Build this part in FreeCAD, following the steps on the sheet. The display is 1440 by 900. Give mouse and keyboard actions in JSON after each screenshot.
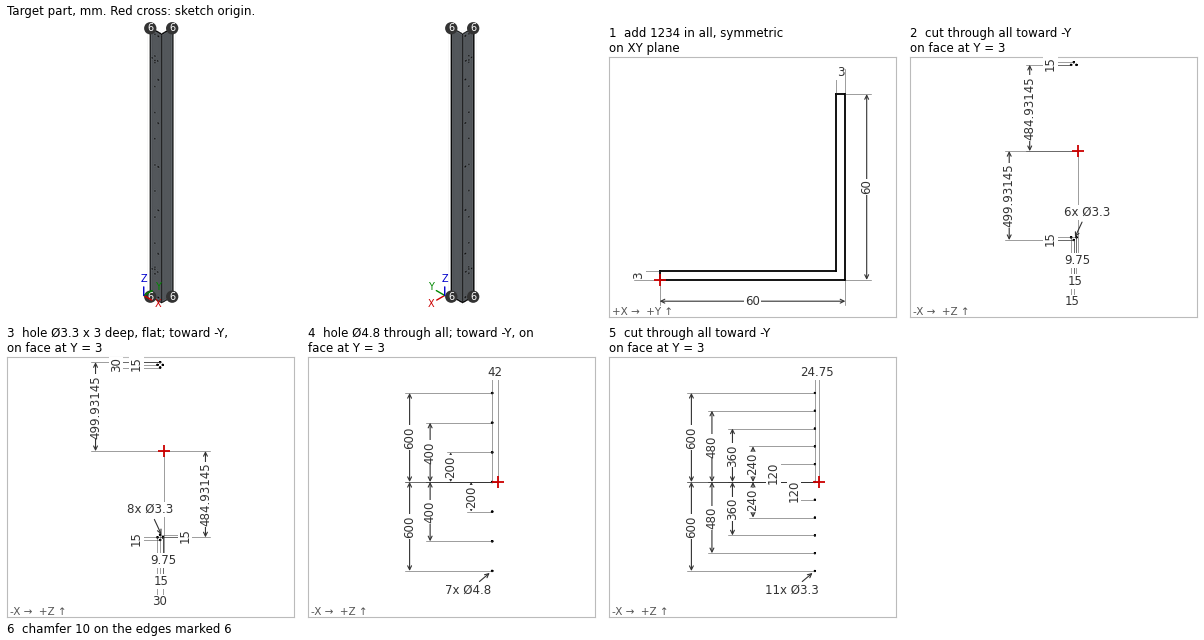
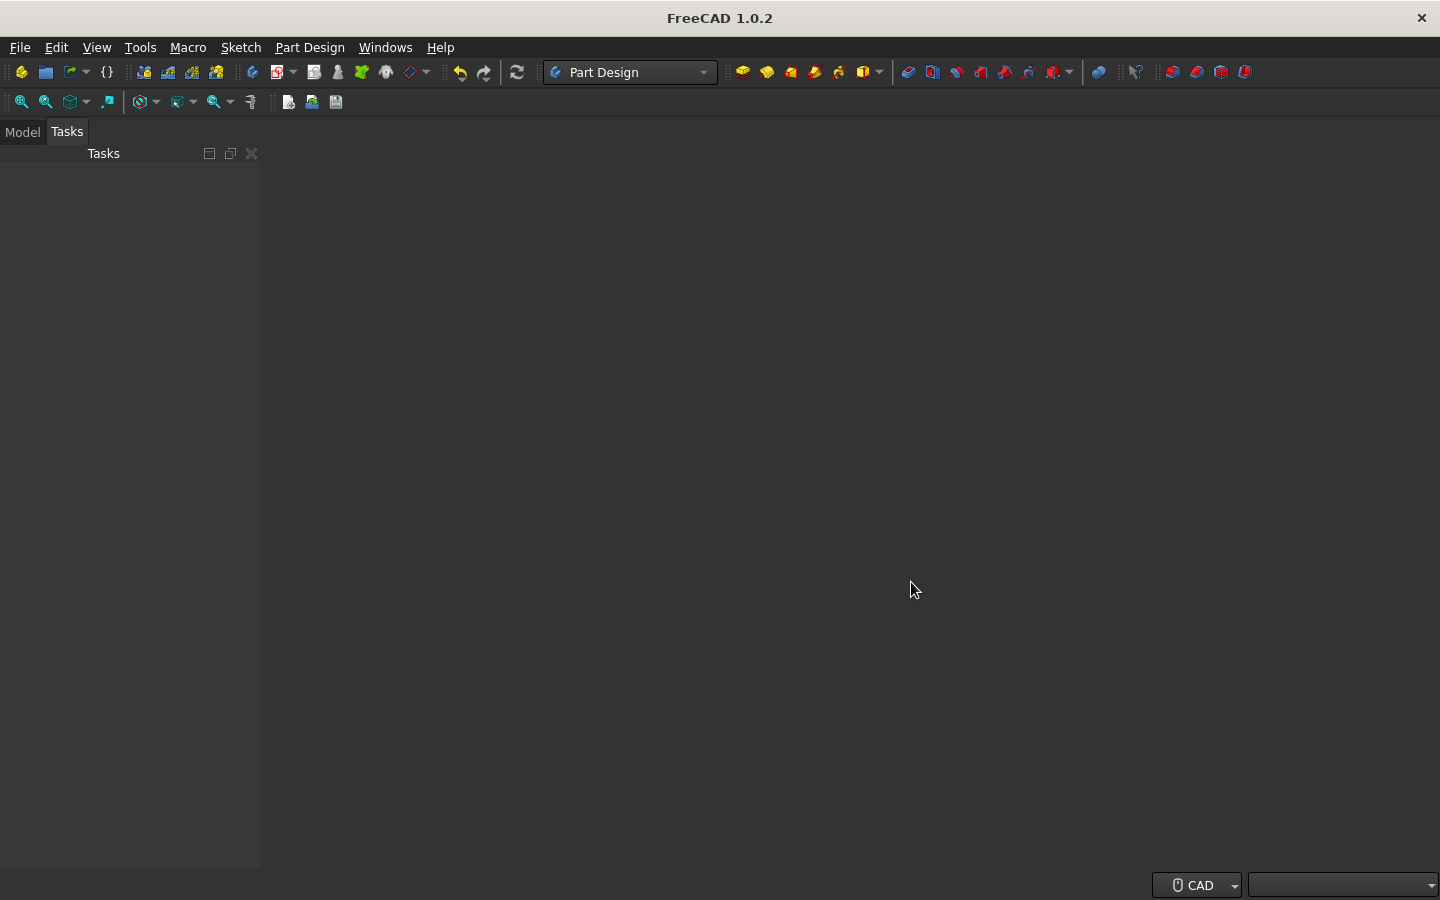
{"action": "left_click", "coordinate": [288, 102]}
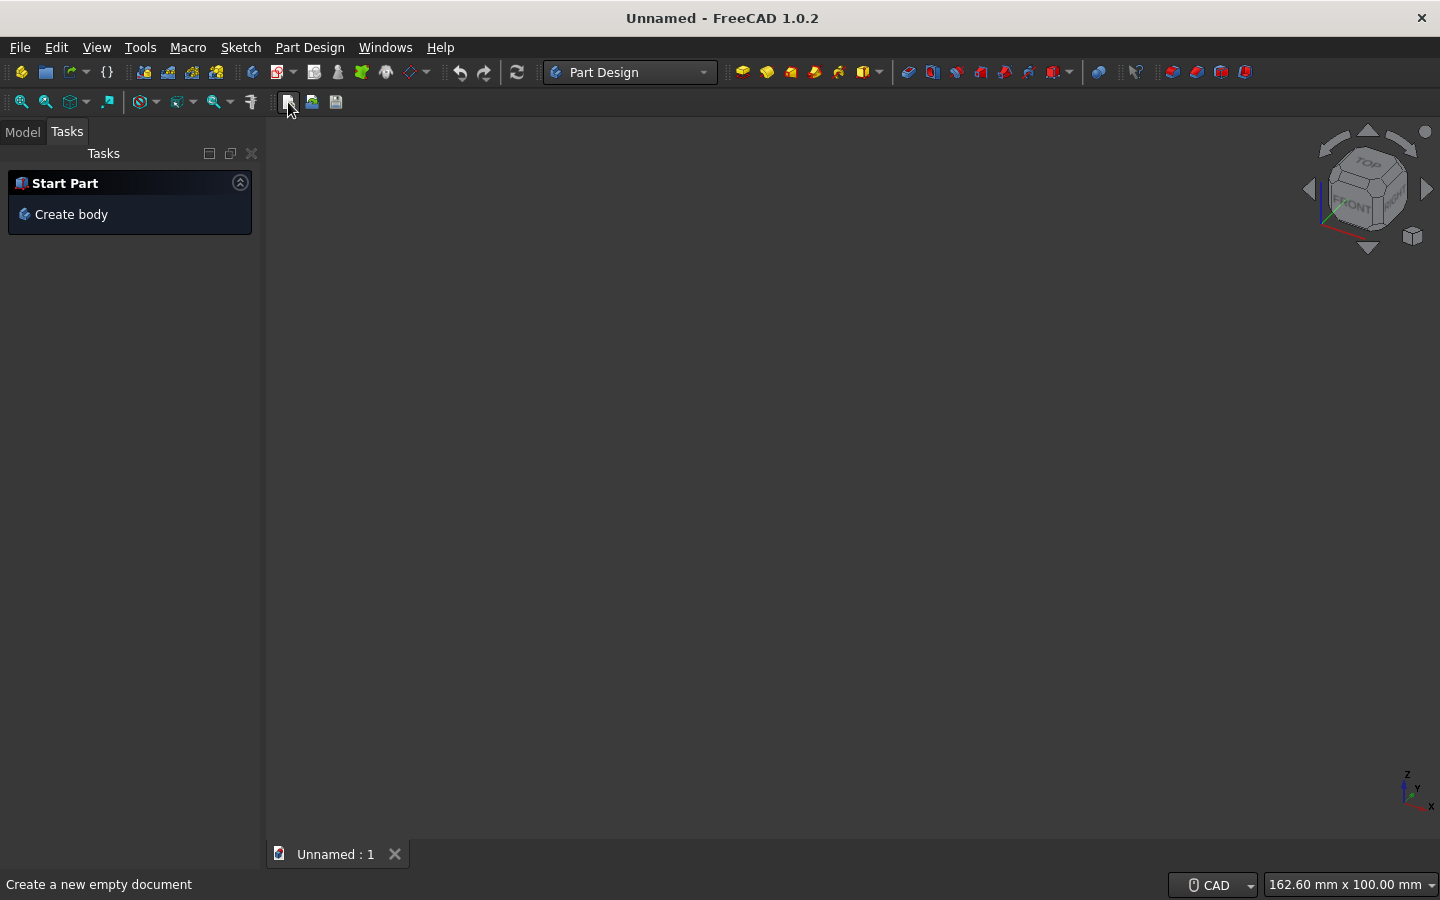
{"action": "left_click", "coordinate": [278, 72]}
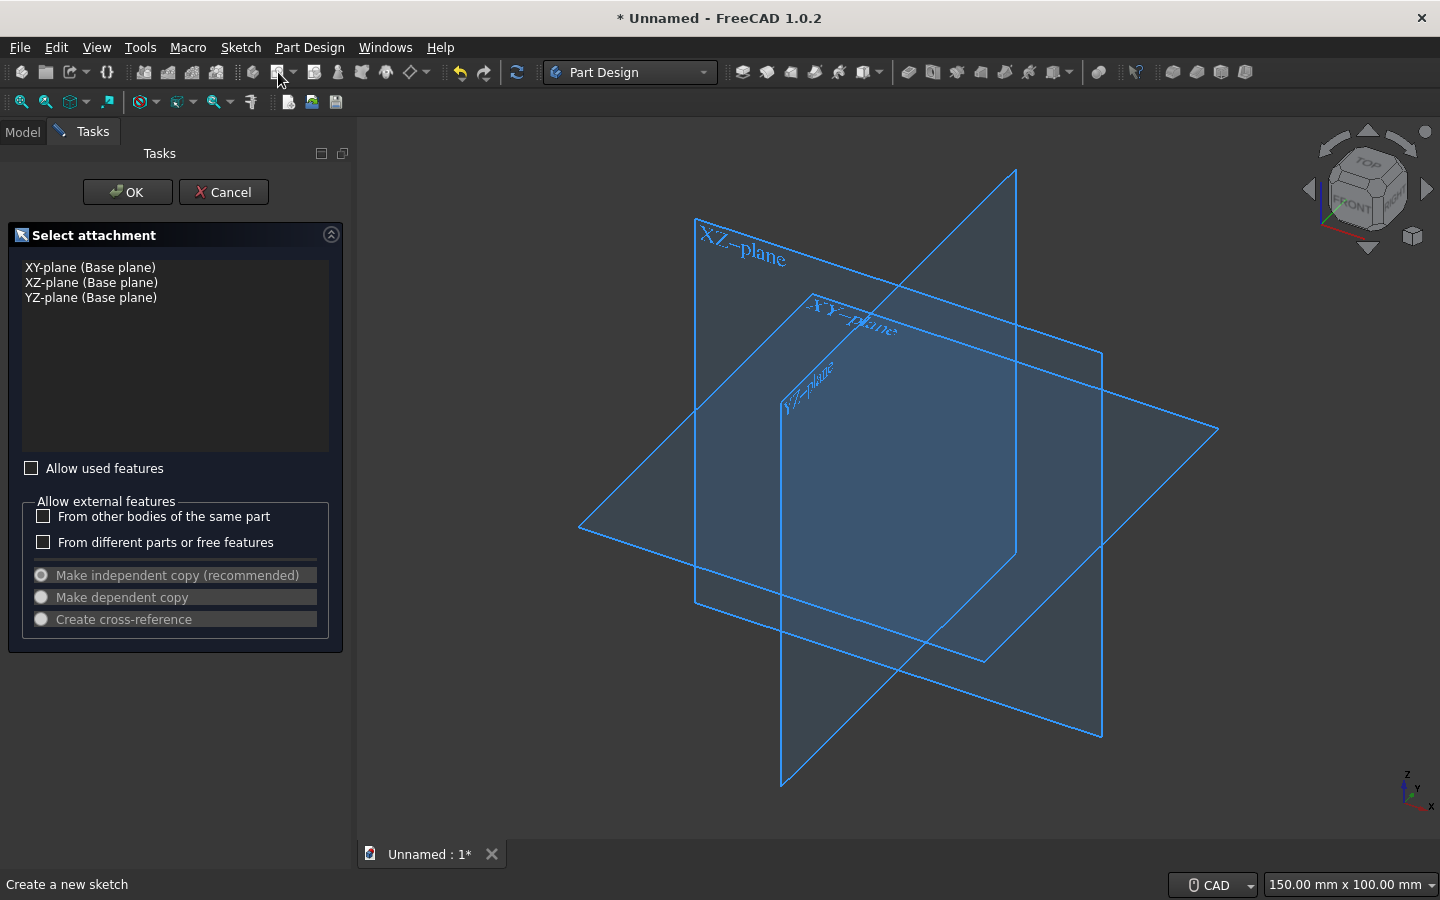
{"action": "left_click", "coordinate": [82, 268]}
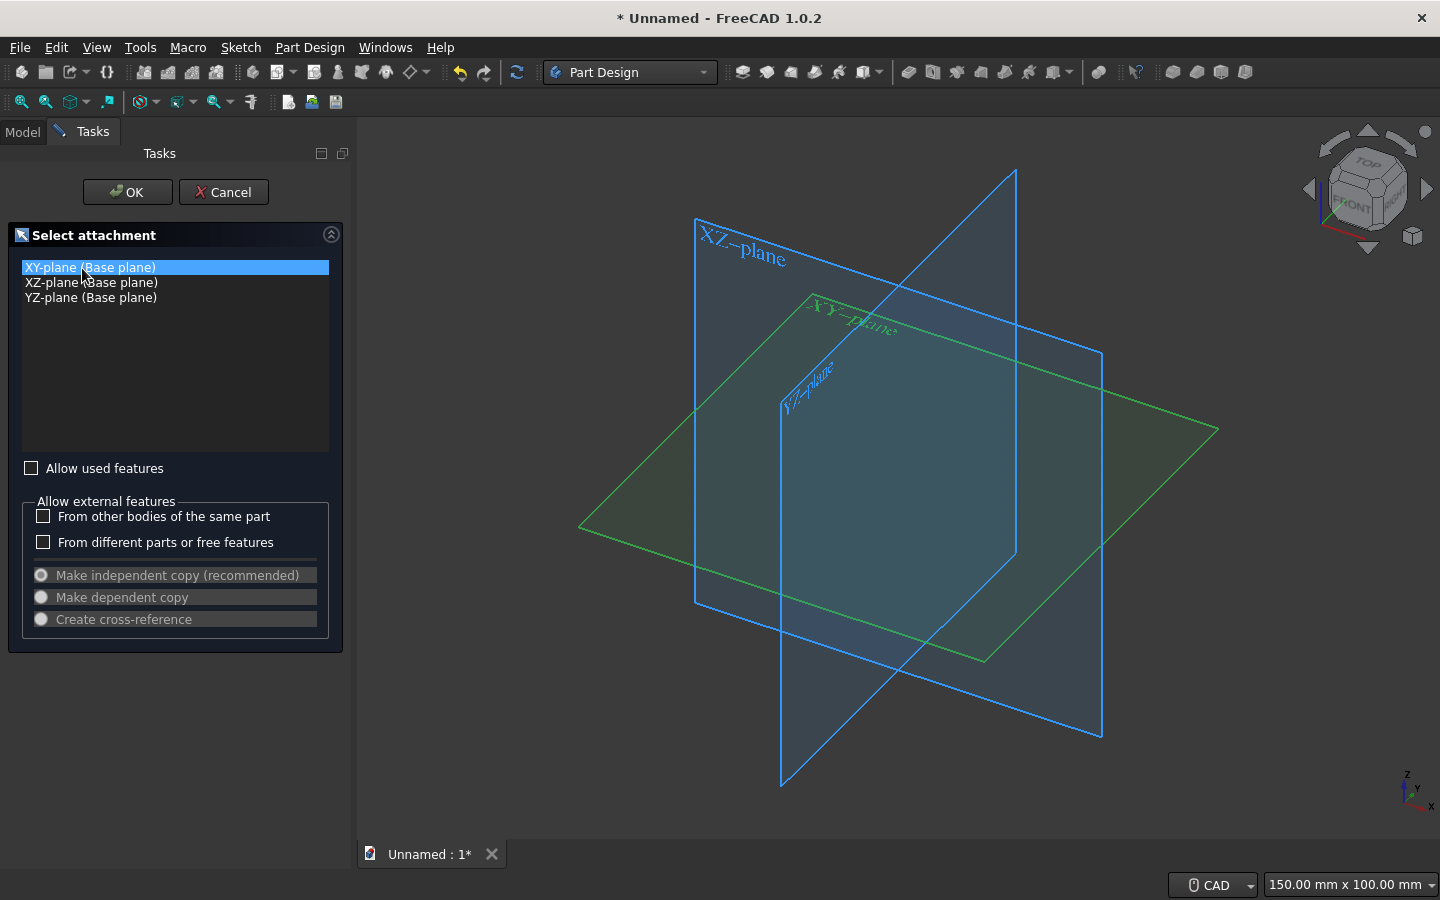
{"action": "left_click", "coordinate": [128, 192]}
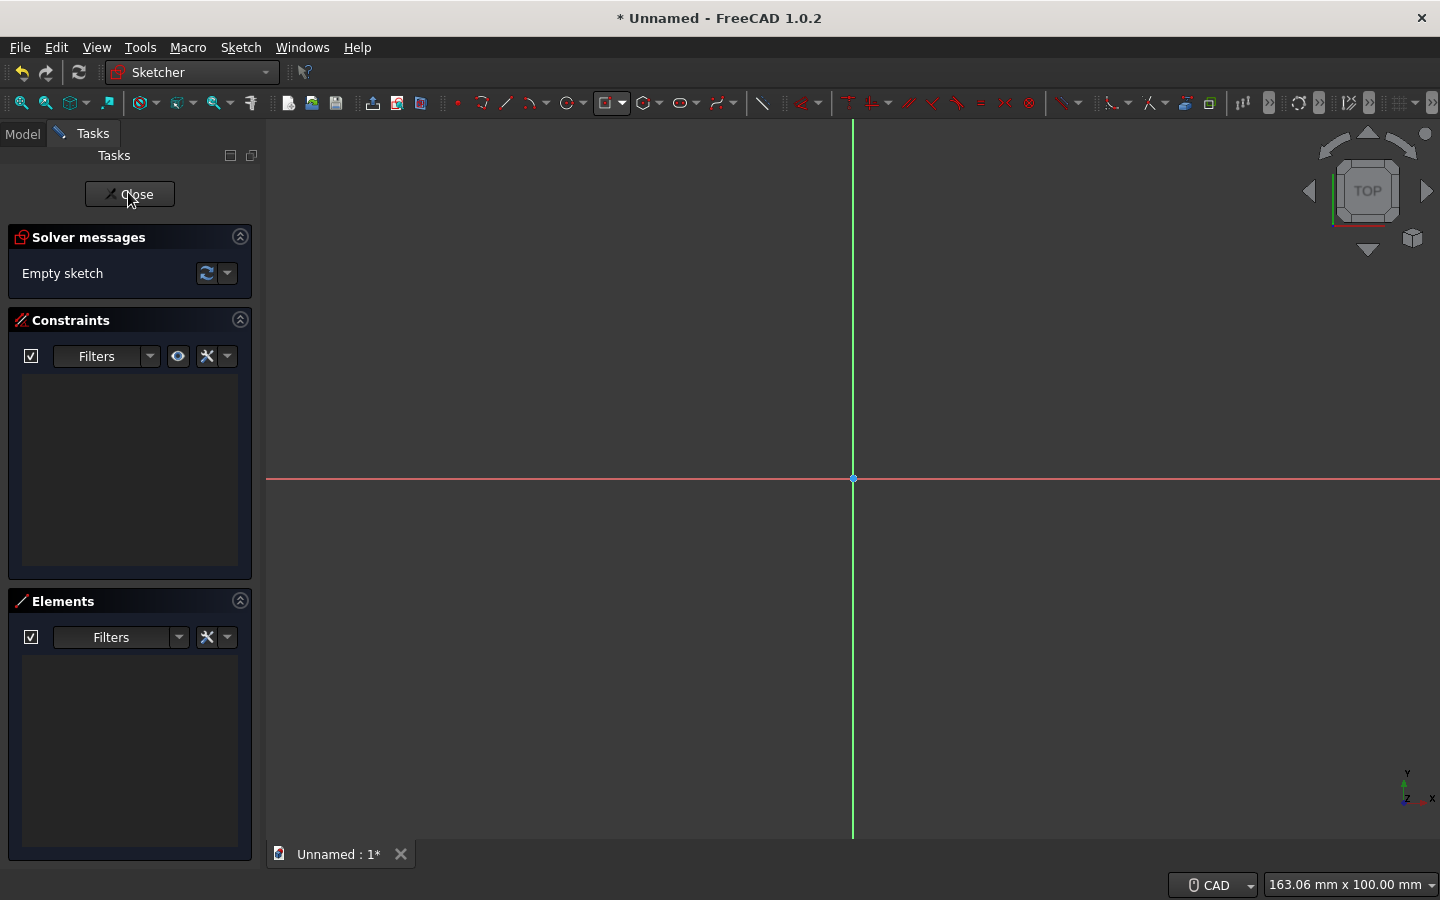
{"action": "scroll", "coordinate": [294, 811], "scroll_direction": "down", "scroll_amount": 1}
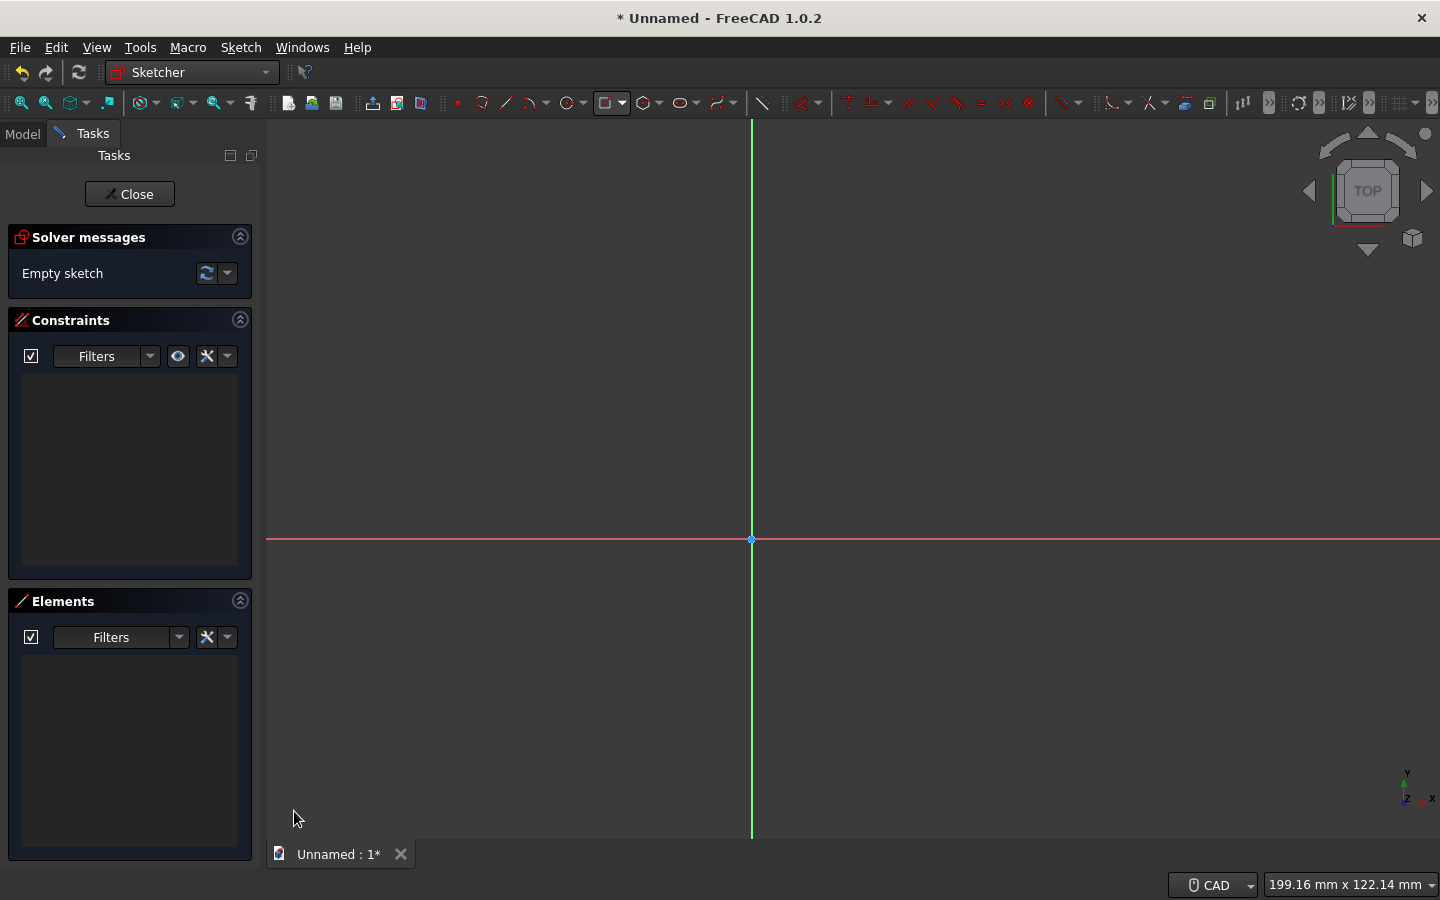
{"action": "left_click", "coordinate": [482, 104]}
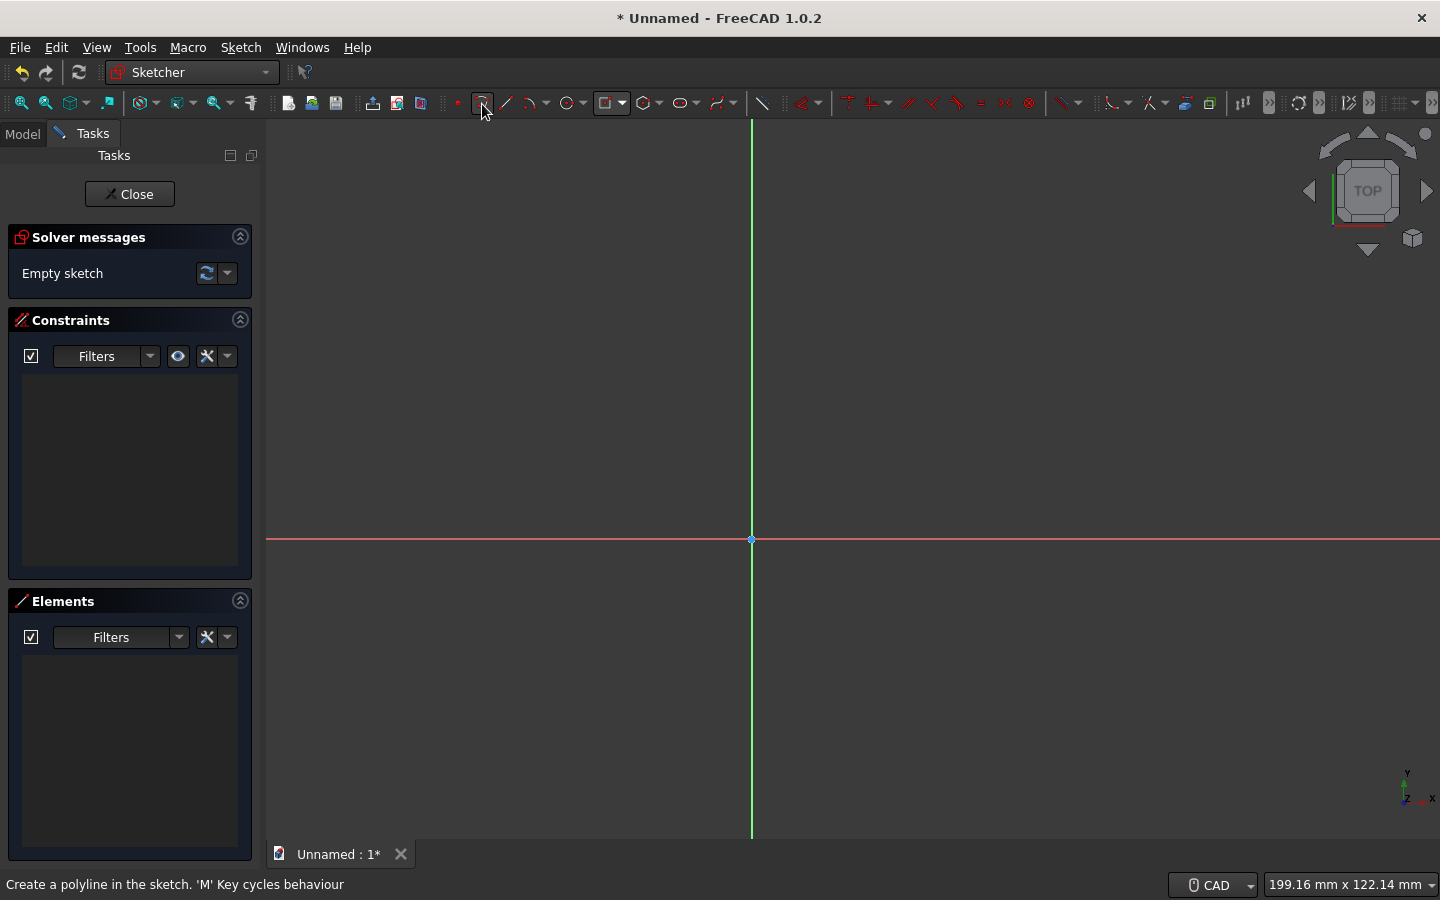
{"action": "left_click", "coordinate": [752, 539]}
{"action": "left_click", "coordinate": [1105, 530]}
{"action": "left_click", "coordinate": [1105, 186]}
{"action": "left_click", "coordinate": [1088, 186]}
{"action": "left_click", "coordinate": [1088, 522]}
{"action": "left_click", "coordinate": [761, 522]}
{"action": "left_click", "coordinate": [752, 539]}
{"action": "key", "text": "Escape"}
{"action": "key", "text": "Escape"}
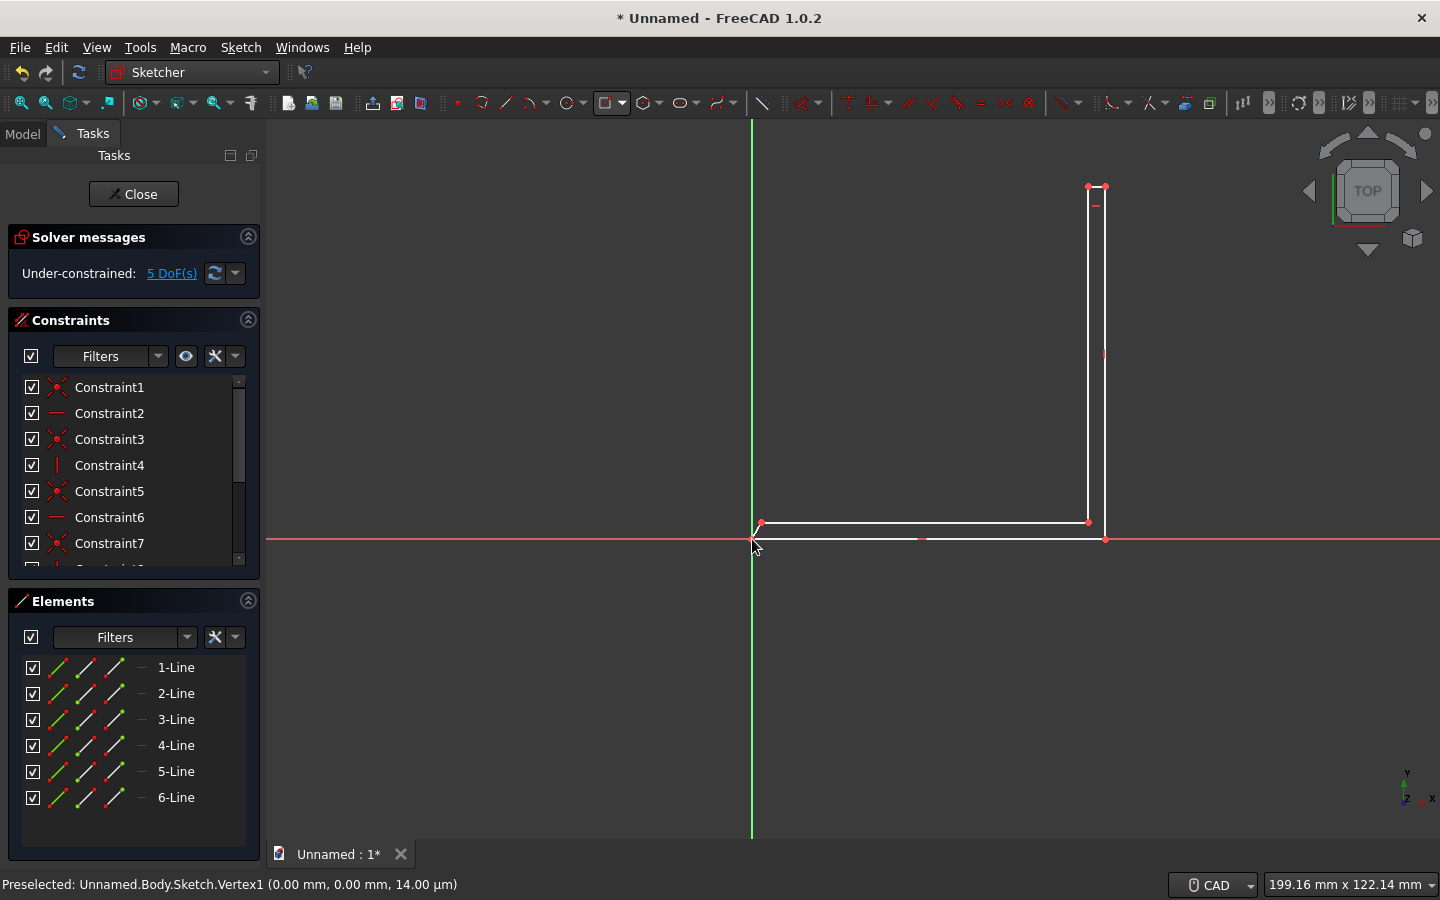
{"action": "scroll", "coordinate": [755, 533], "scroll_direction": "up", "scroll_amount": 4}